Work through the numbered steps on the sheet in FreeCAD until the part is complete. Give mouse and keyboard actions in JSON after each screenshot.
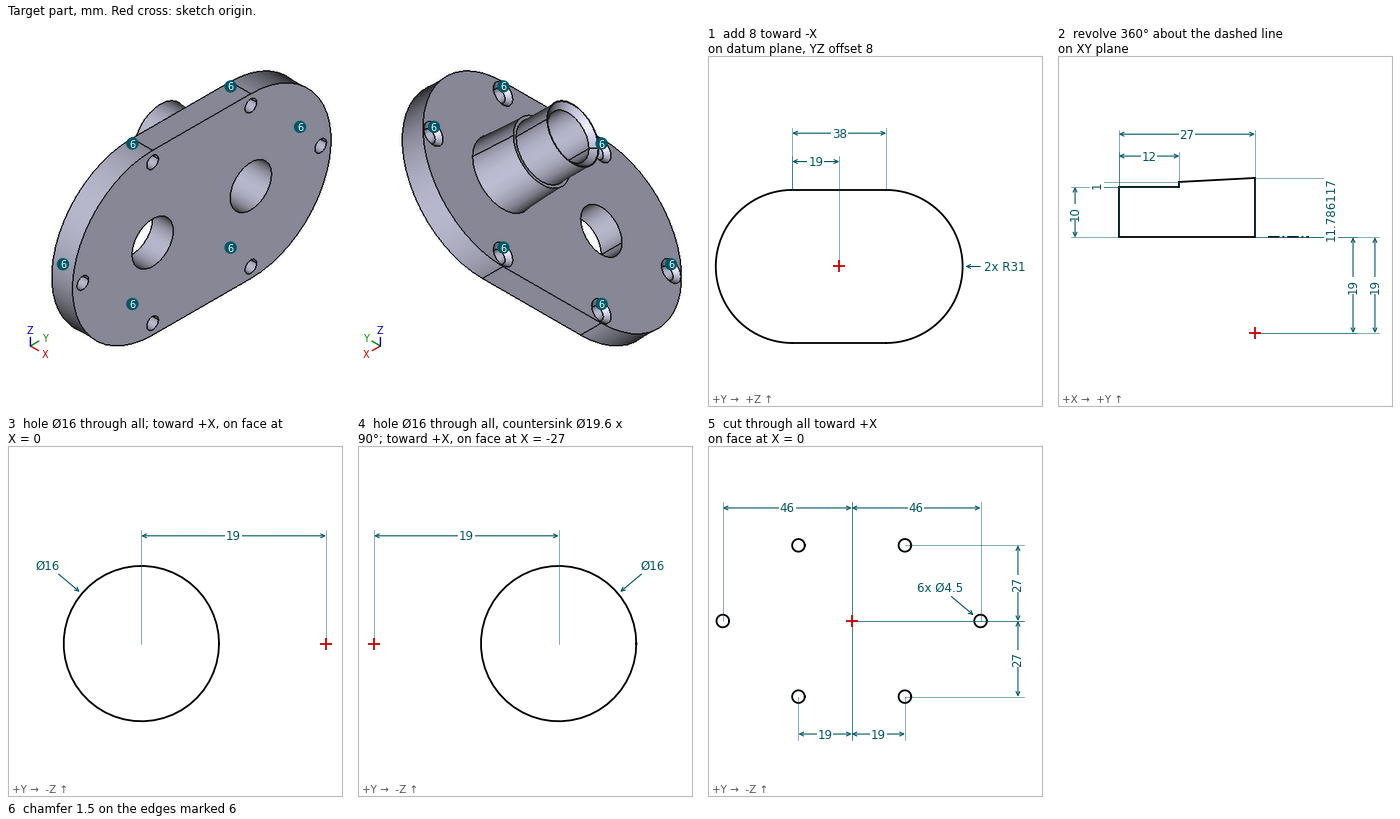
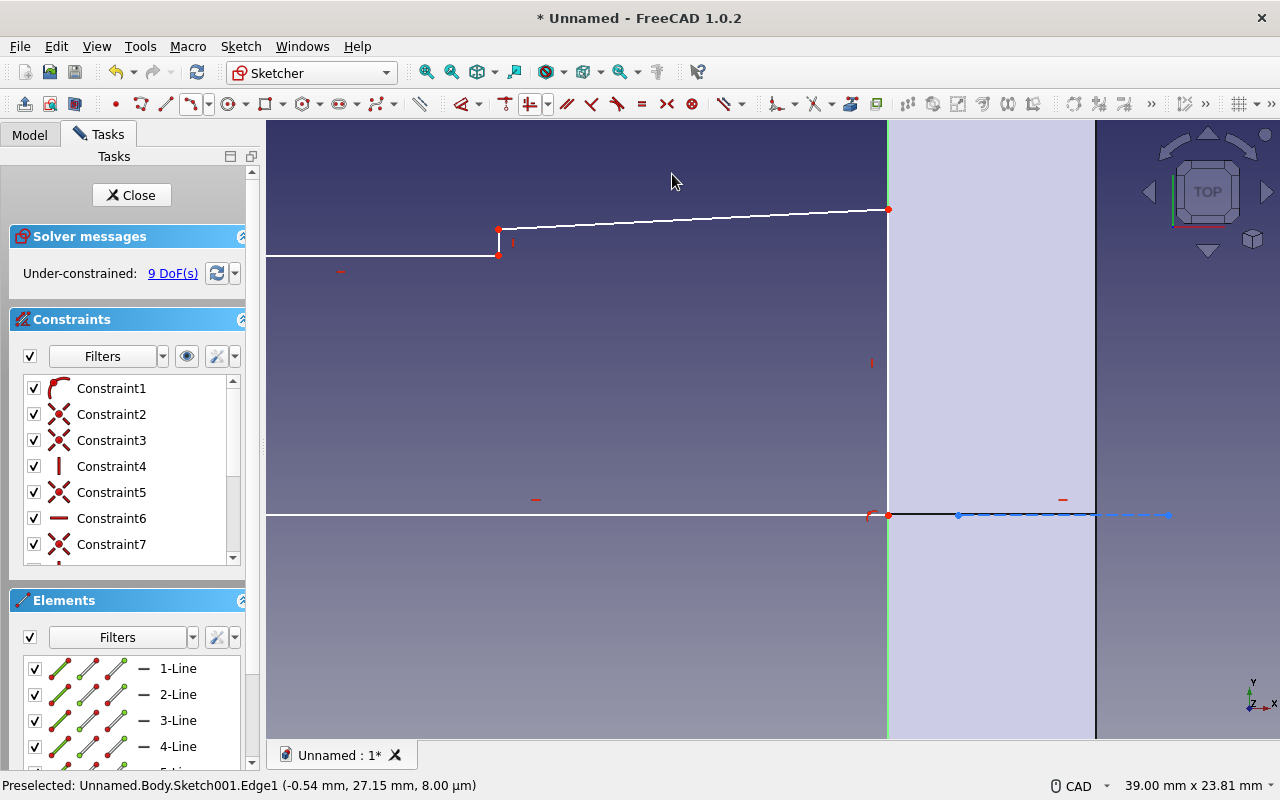
{"action": "key", "text": "d"}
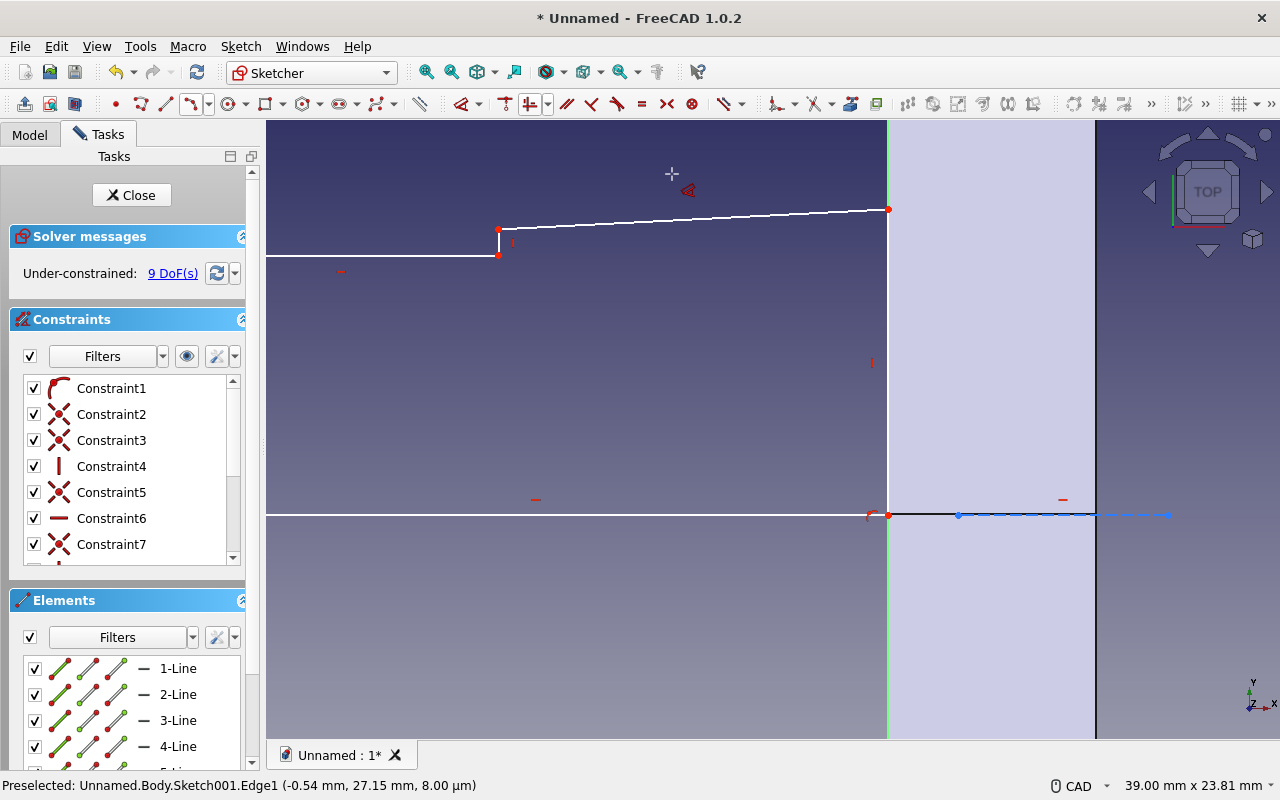
{"action": "scroll", "coordinate": [499, 240], "scroll_direction": "up", "scroll_amount": 3}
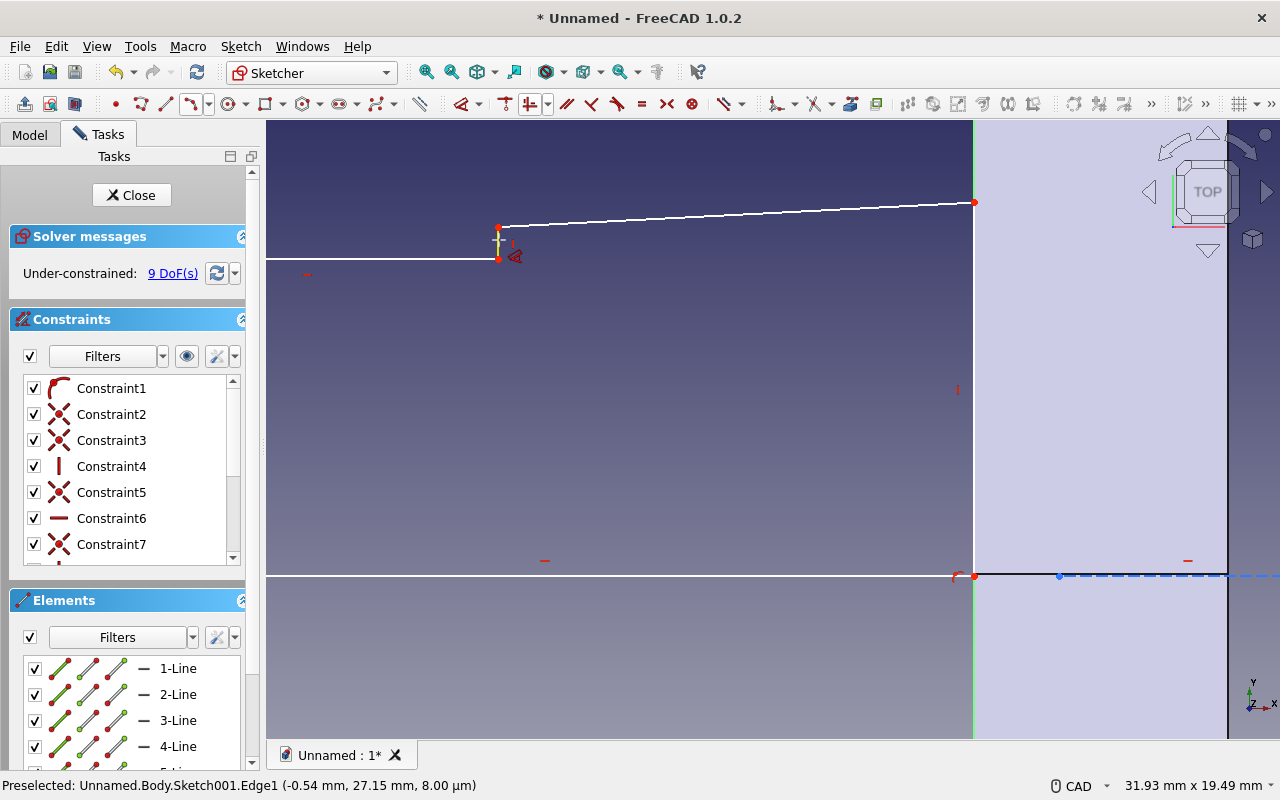
{"action": "left_click", "coordinate": [498, 240]}
{"action": "left_click", "coordinate": [464, 244]}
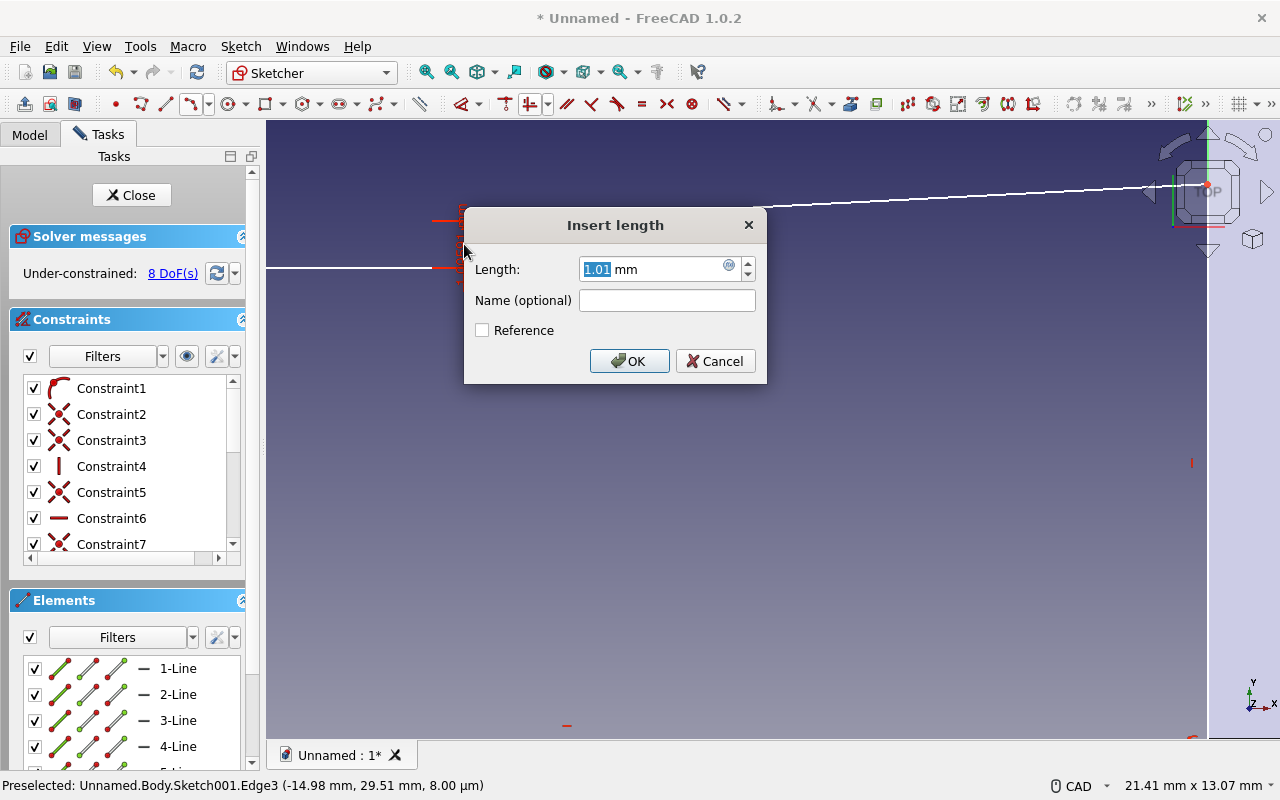
{"action": "type", "text": "1"}
{"action": "key", "text": "Return"}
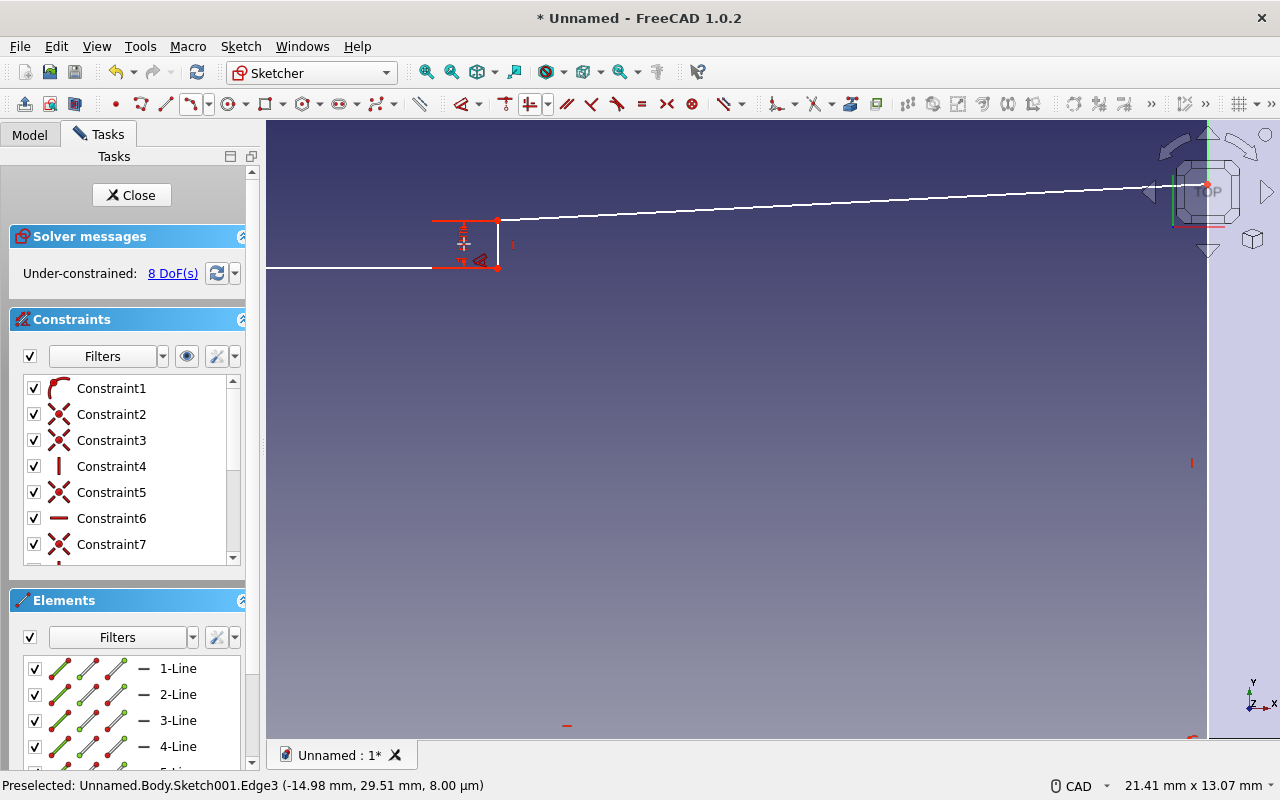
{"action": "scroll", "coordinate": [665, 272], "scroll_direction": "down", "scroll_amount": 7}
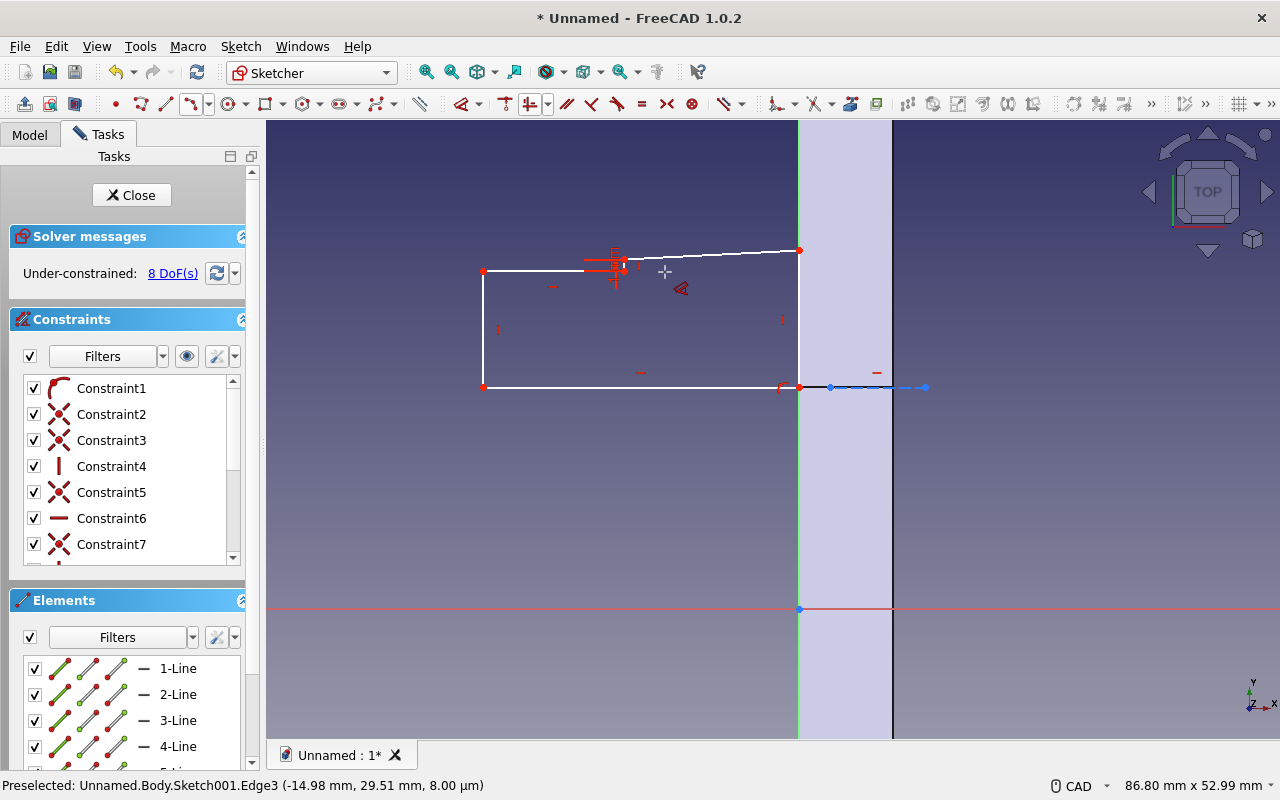
{"action": "left_click", "coordinate": [582, 271]}
{"action": "left_click", "coordinate": [554, 237]}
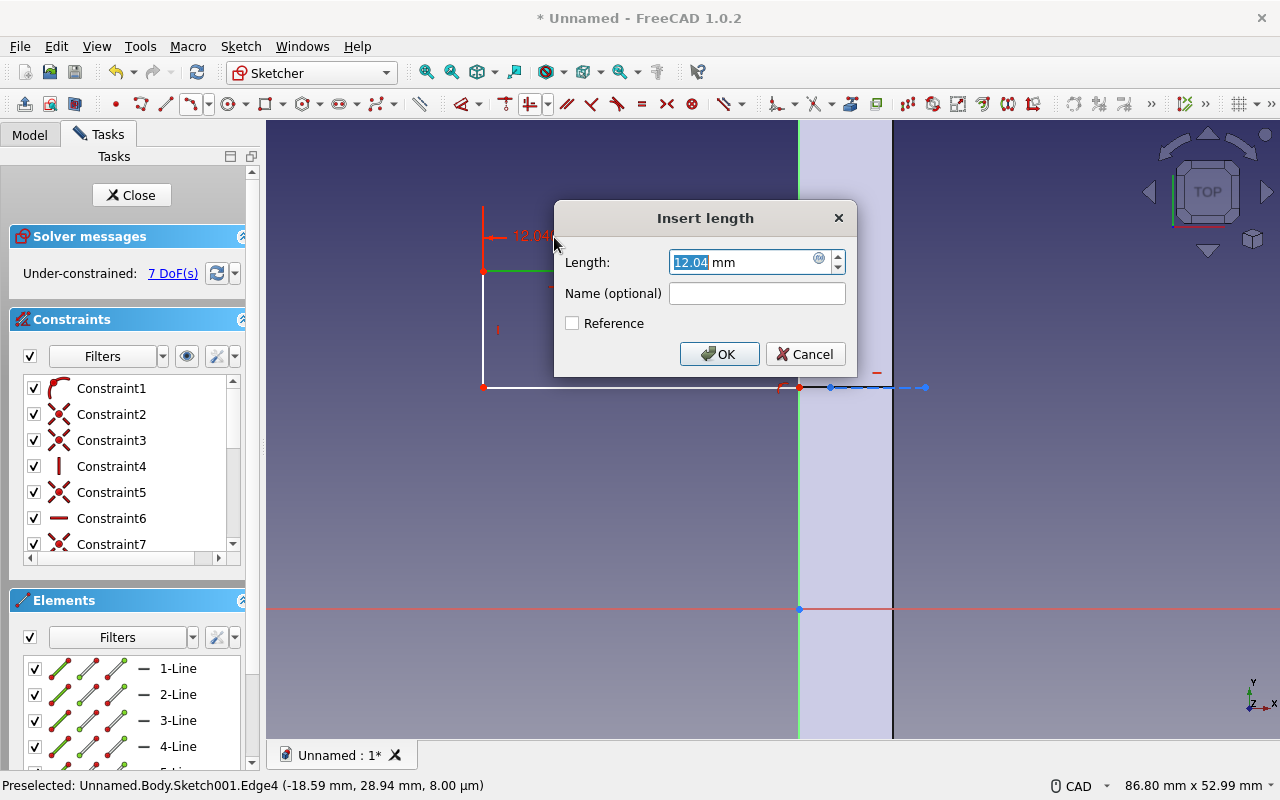
{"action": "type", "text": "12"}
{"action": "key", "text": "Return"}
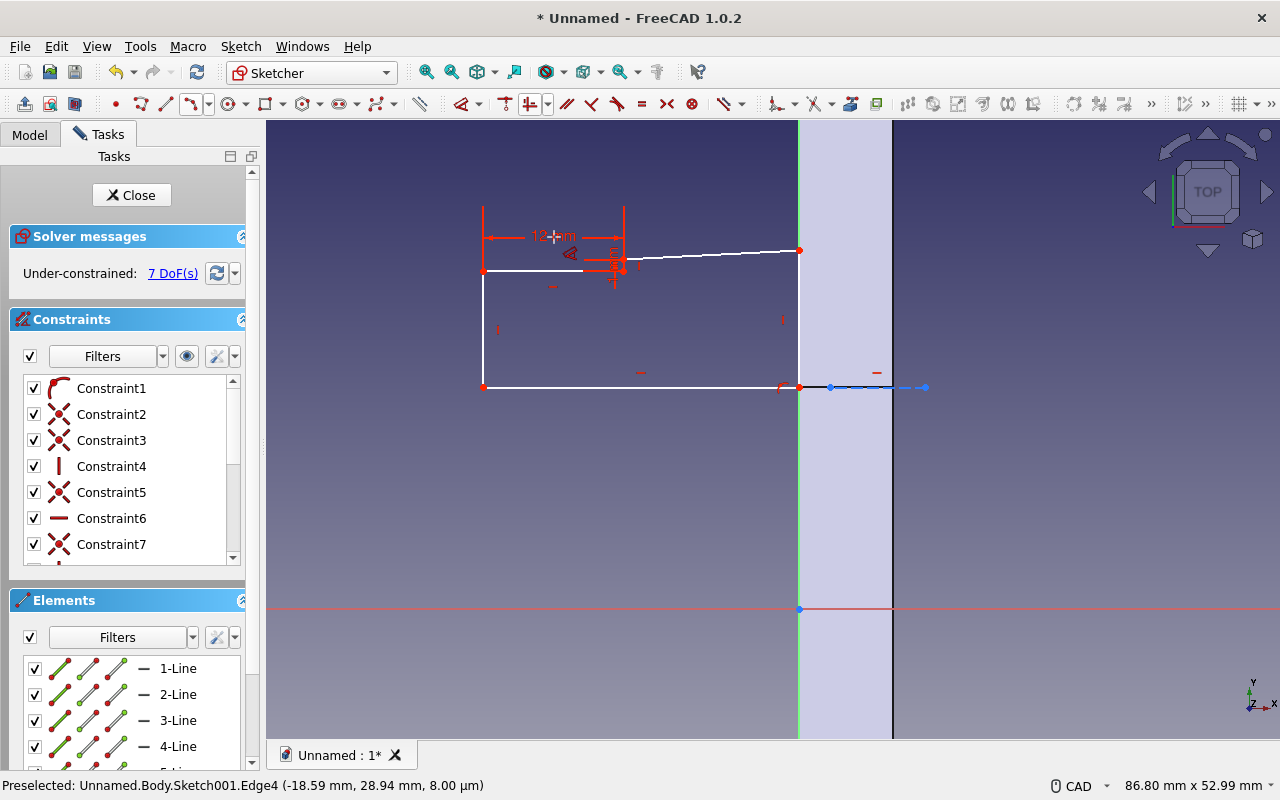
{"action": "left_click", "coordinate": [483, 306]}
{"action": "left_click", "coordinate": [449, 330]}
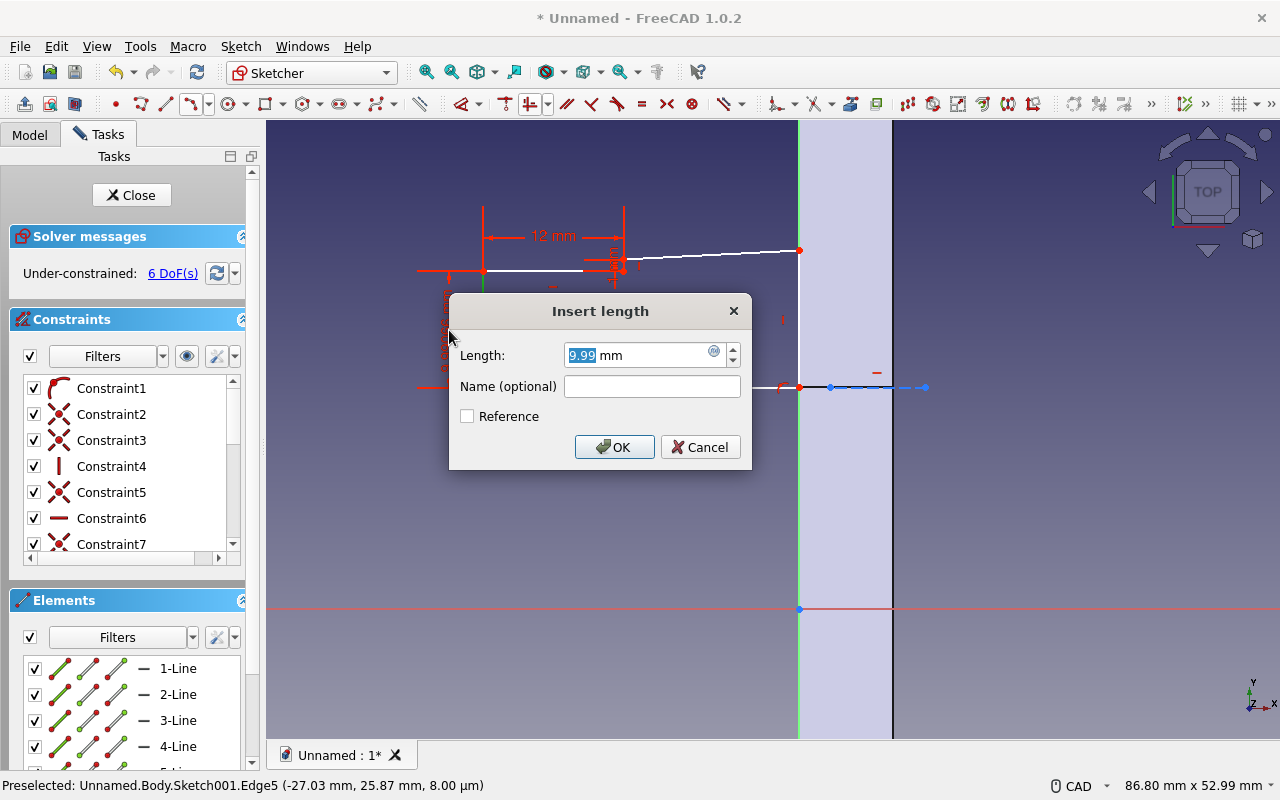
{"action": "type", "text": "10"}
{"action": "key", "text": "Return"}